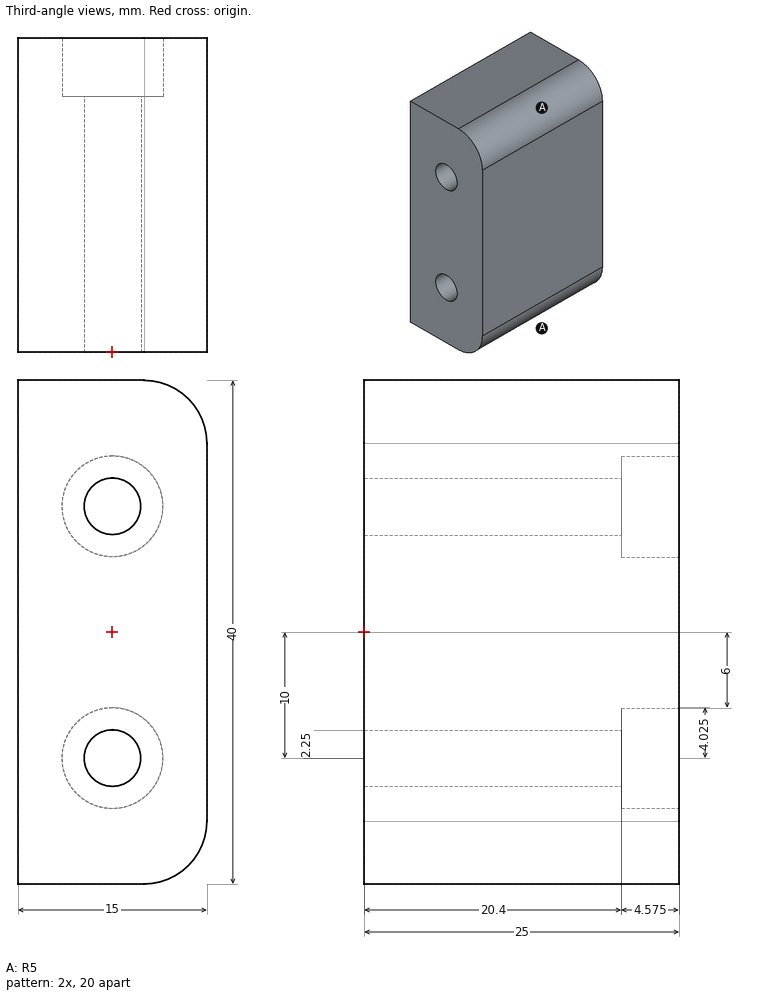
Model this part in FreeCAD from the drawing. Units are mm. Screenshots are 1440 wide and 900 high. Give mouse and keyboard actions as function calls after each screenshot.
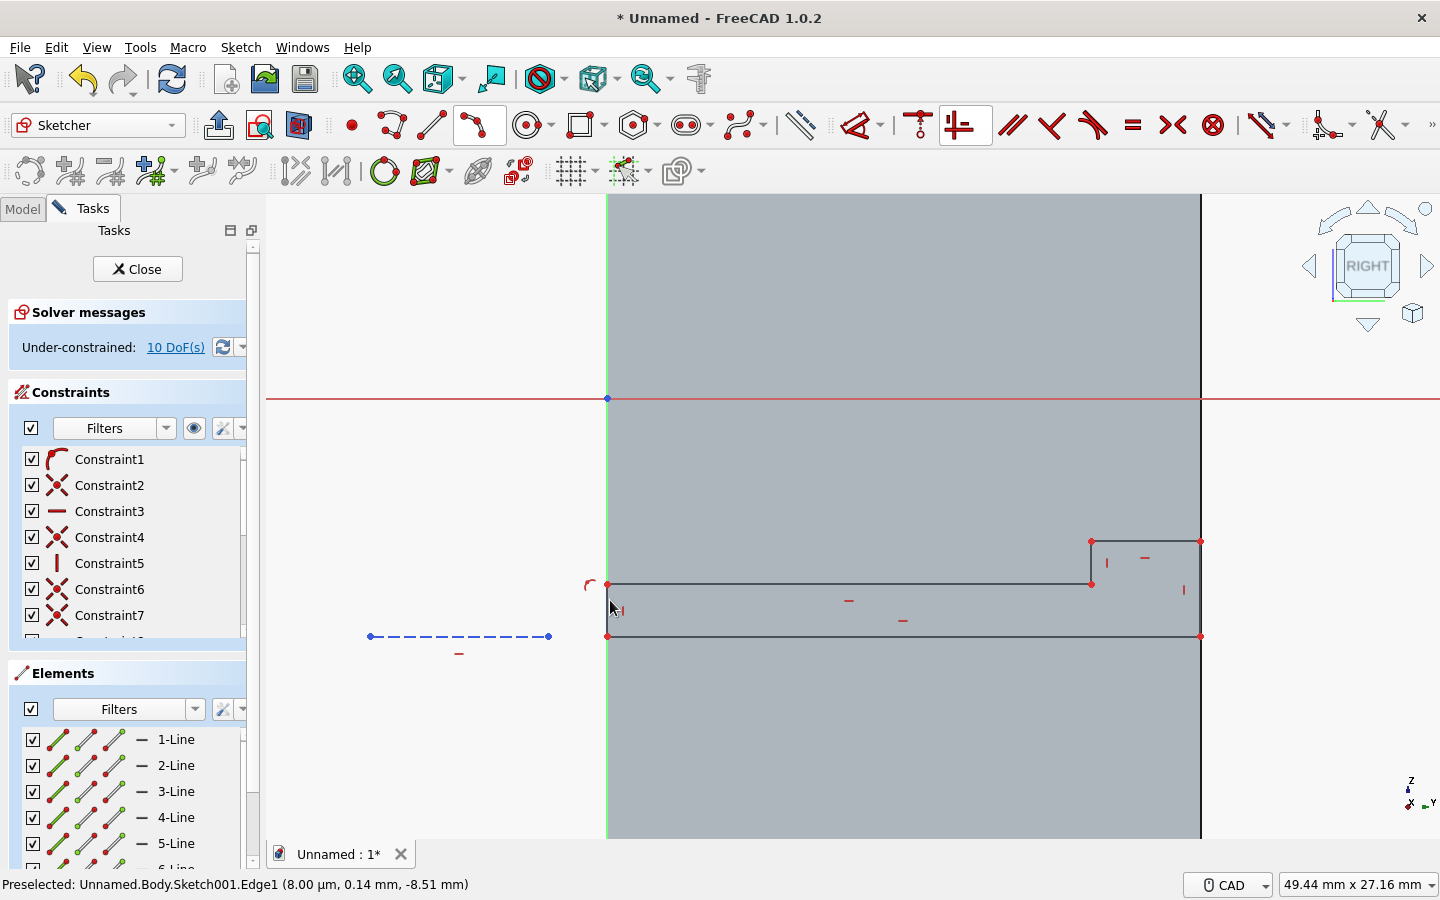
click(856, 126)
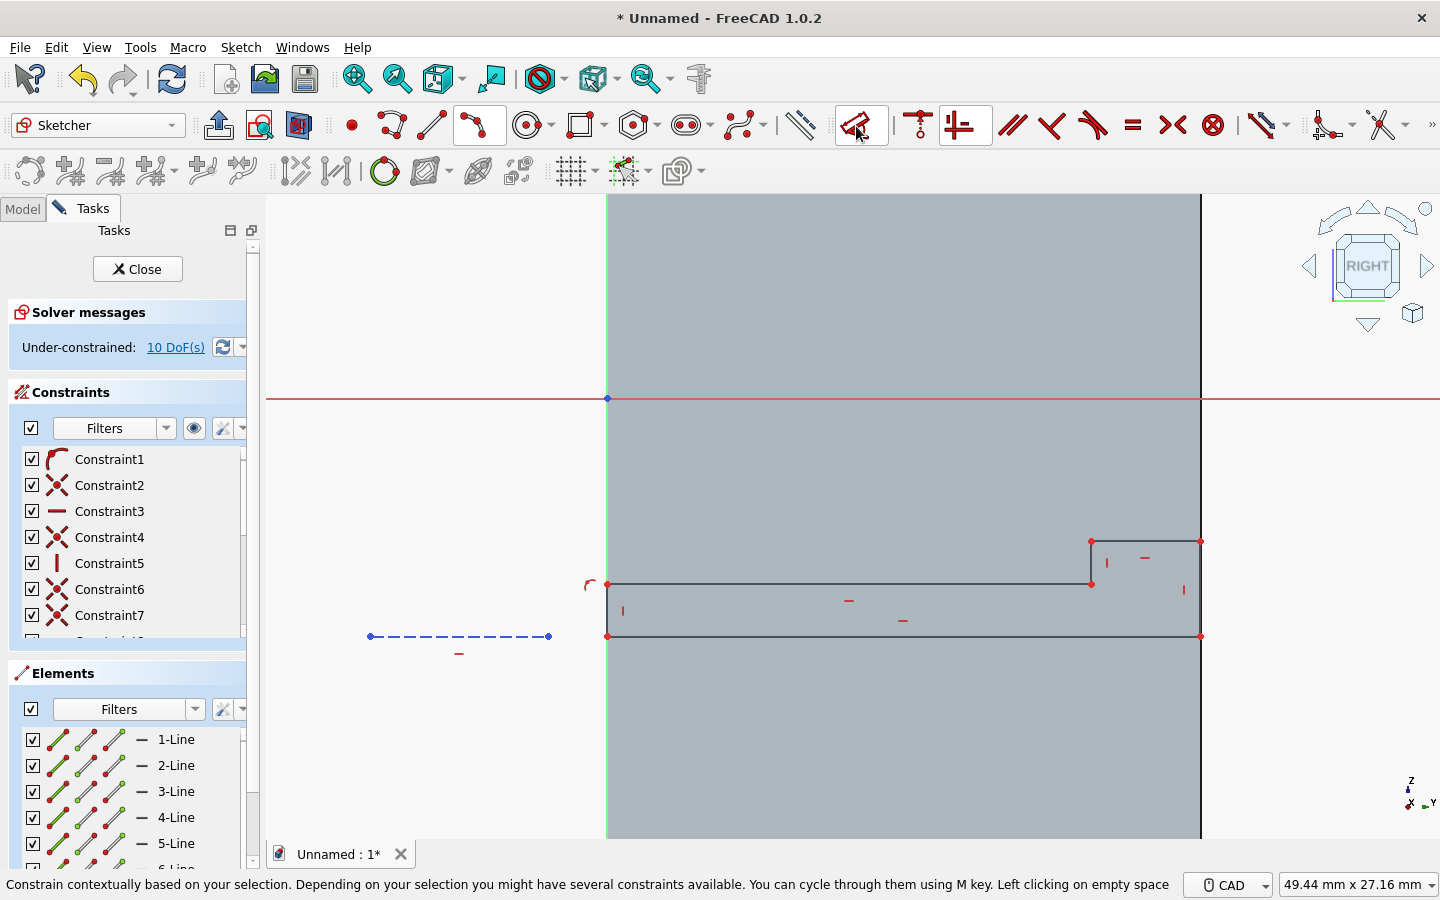
click(785, 637)
click(904, 671)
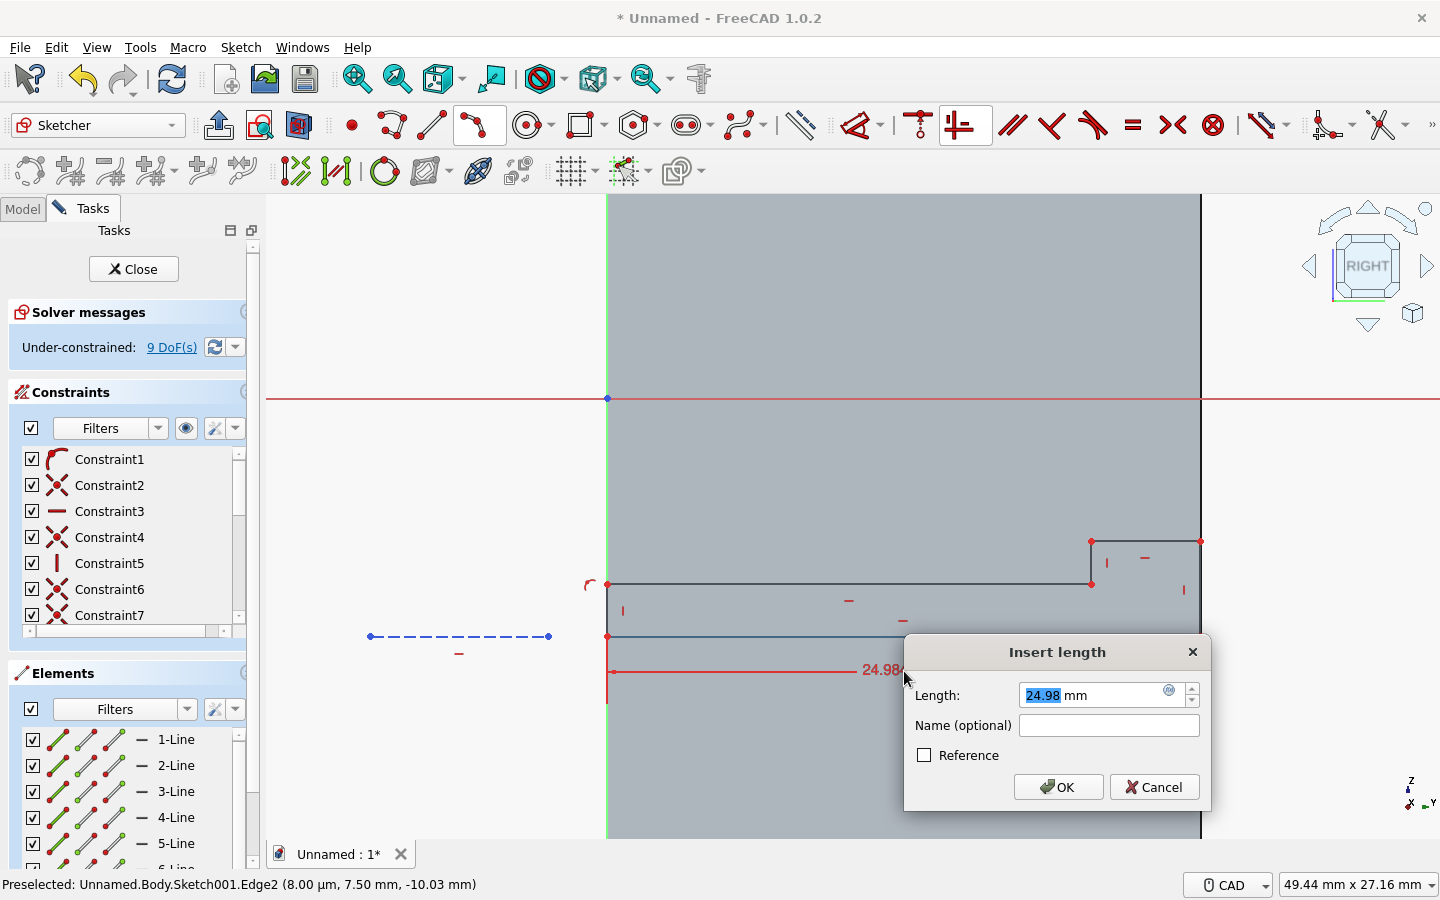
text(25)
key(Return)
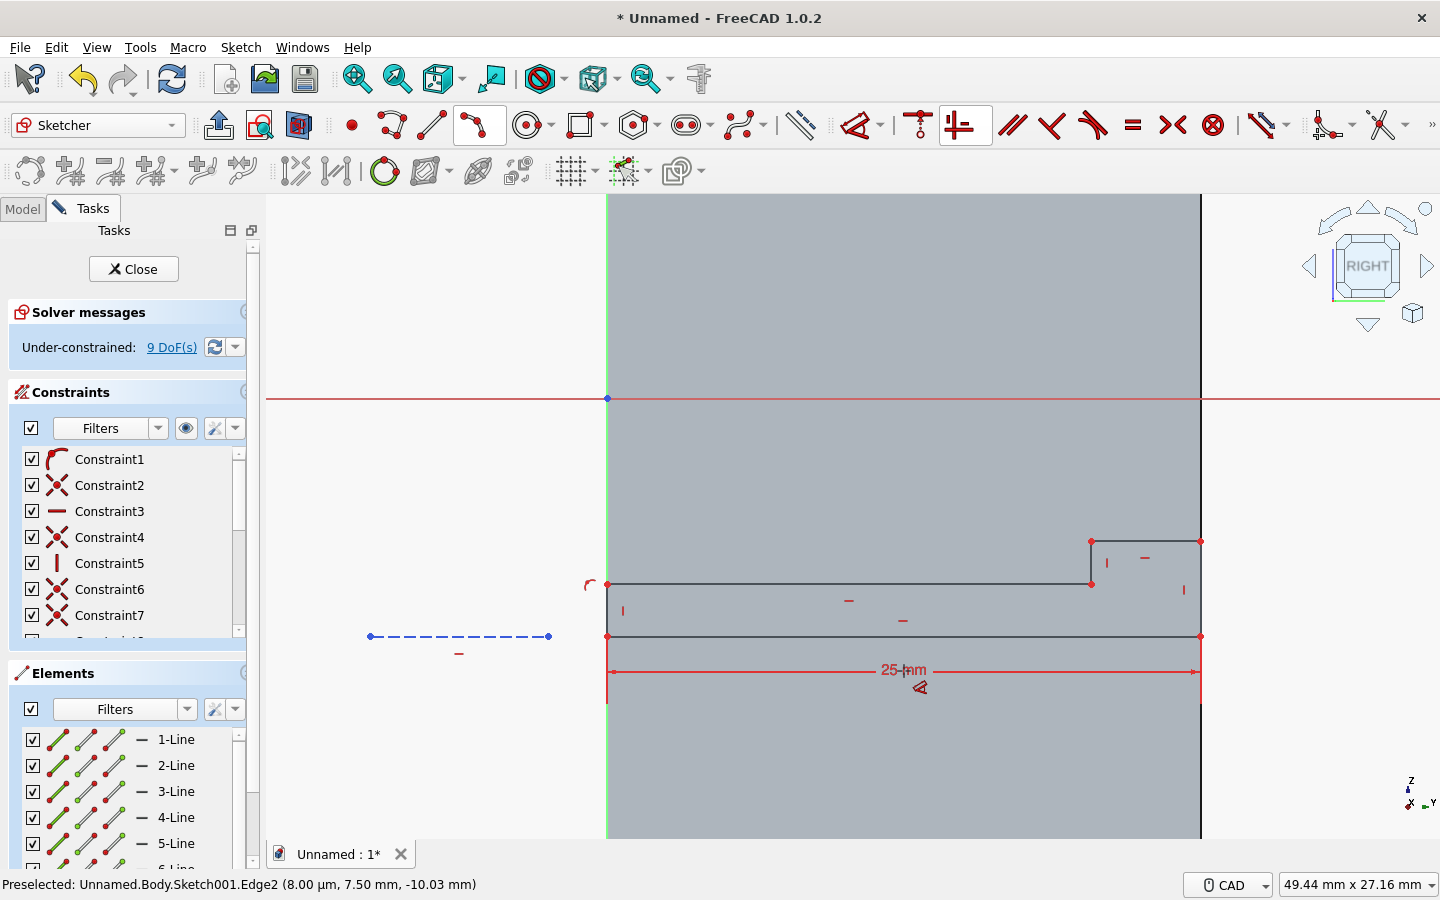
scroll(1200, 541, up, 13)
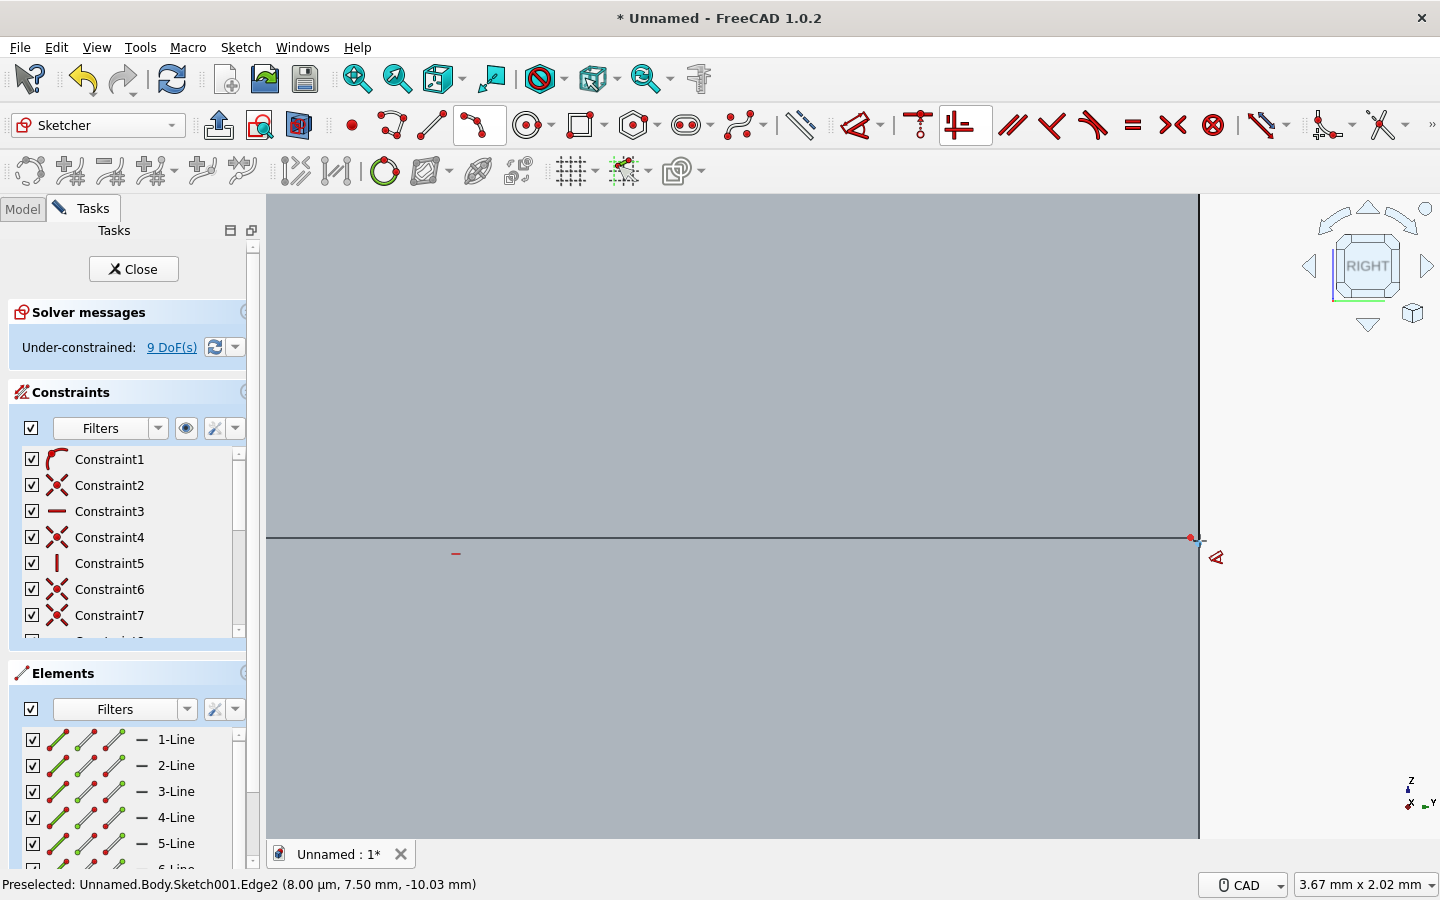
click(1191, 538)
click(1225, 380)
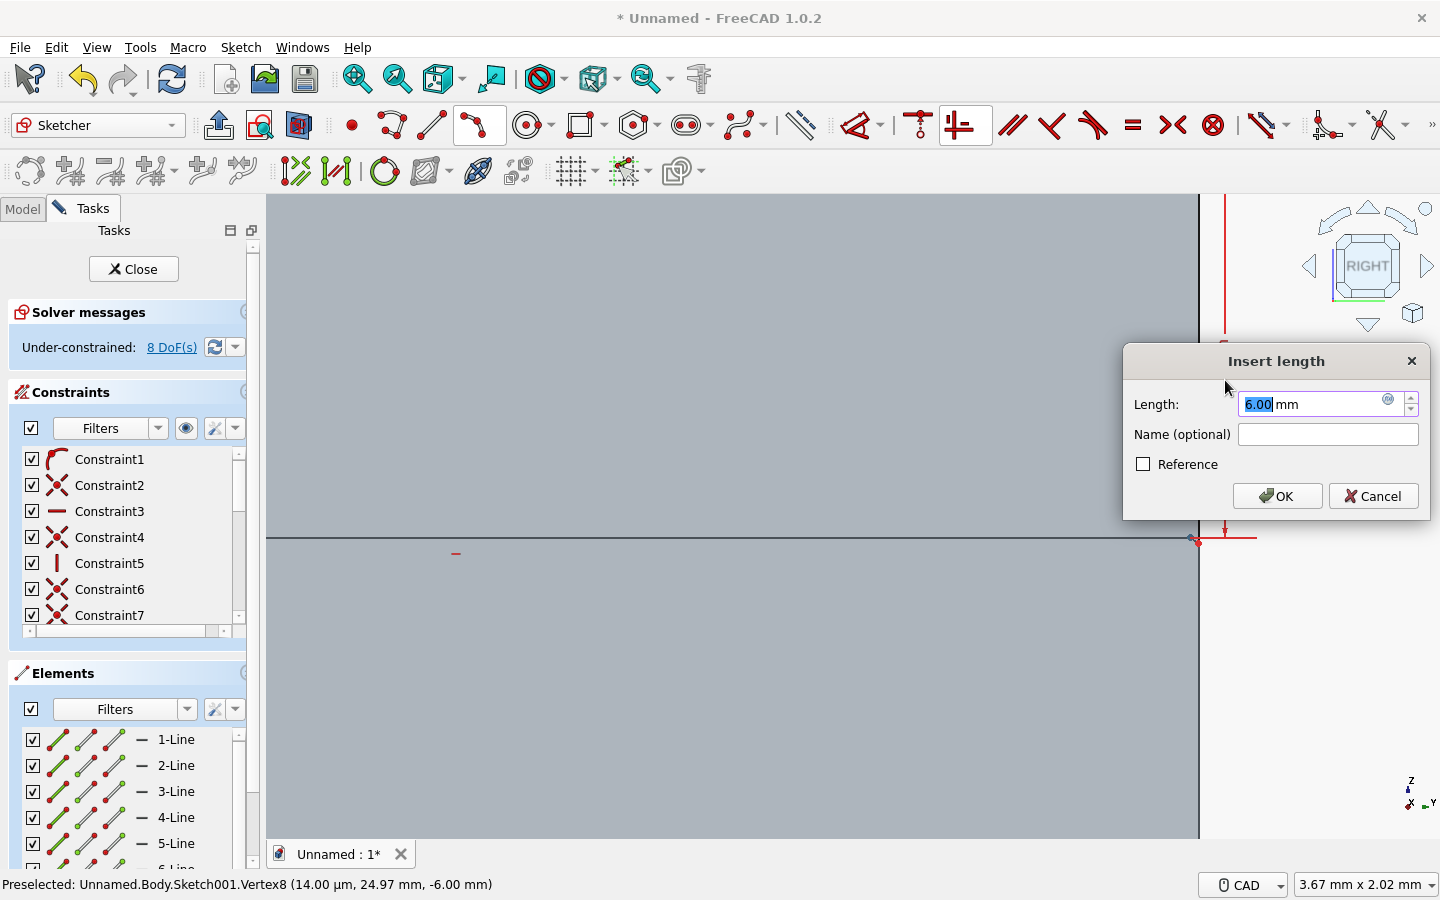
text(6)
key(Return)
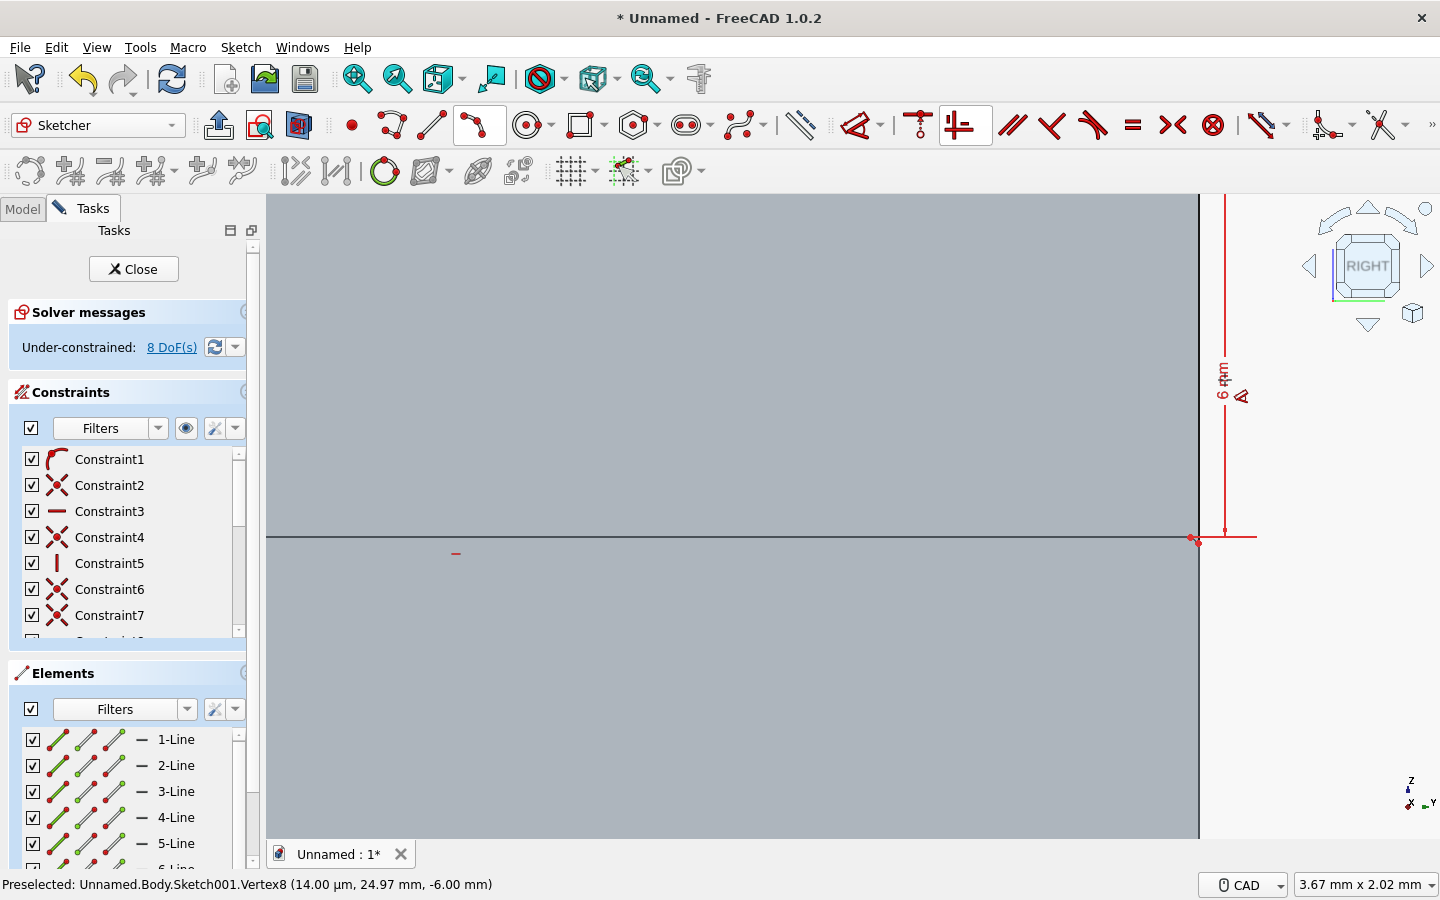
scroll(1120, 536, down, 14)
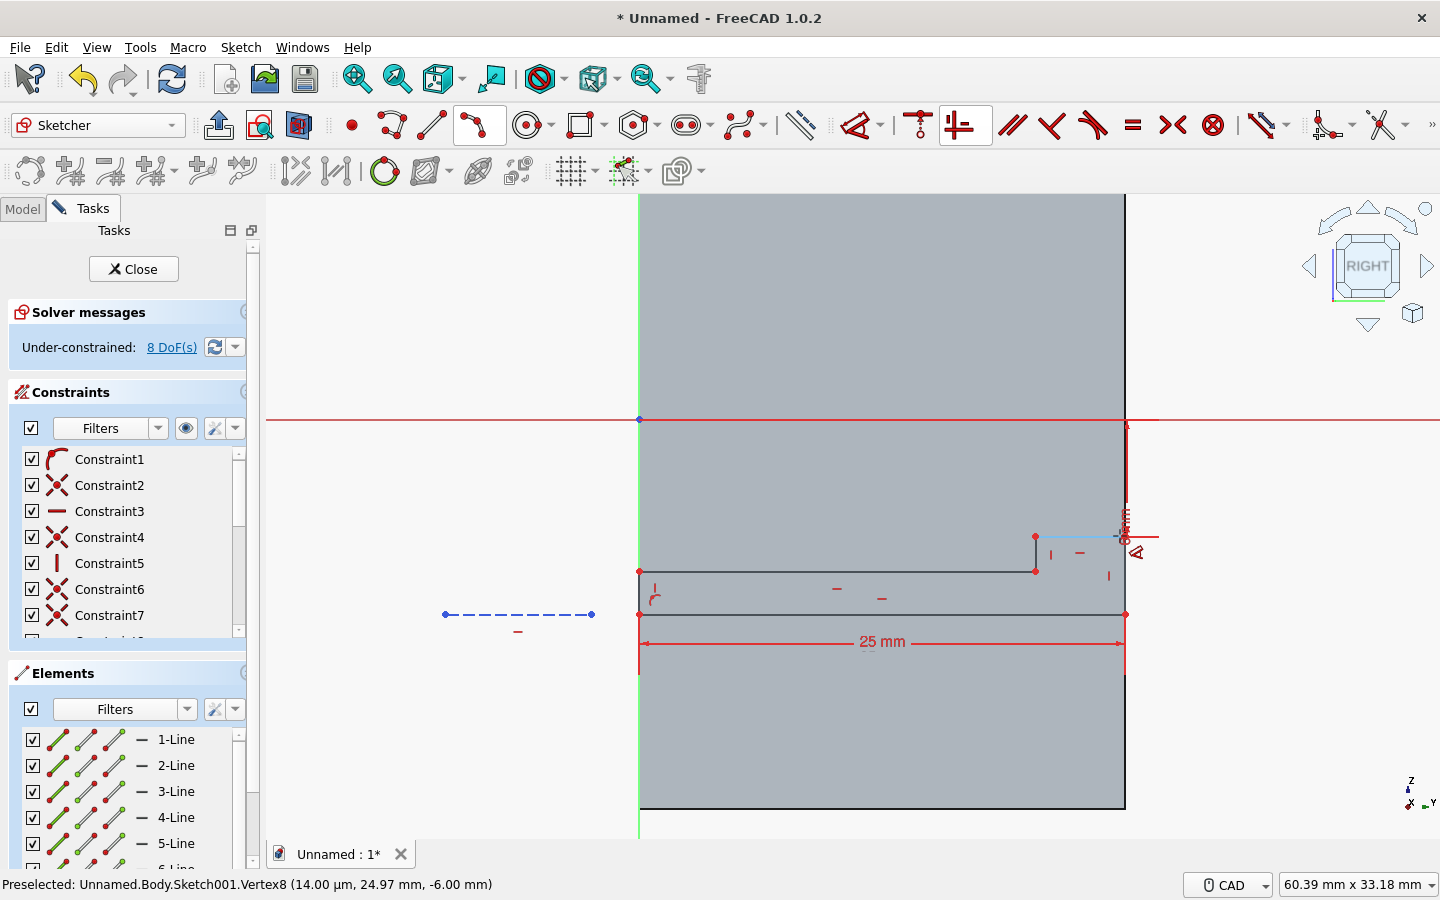
click(639, 615)
click(605, 517)